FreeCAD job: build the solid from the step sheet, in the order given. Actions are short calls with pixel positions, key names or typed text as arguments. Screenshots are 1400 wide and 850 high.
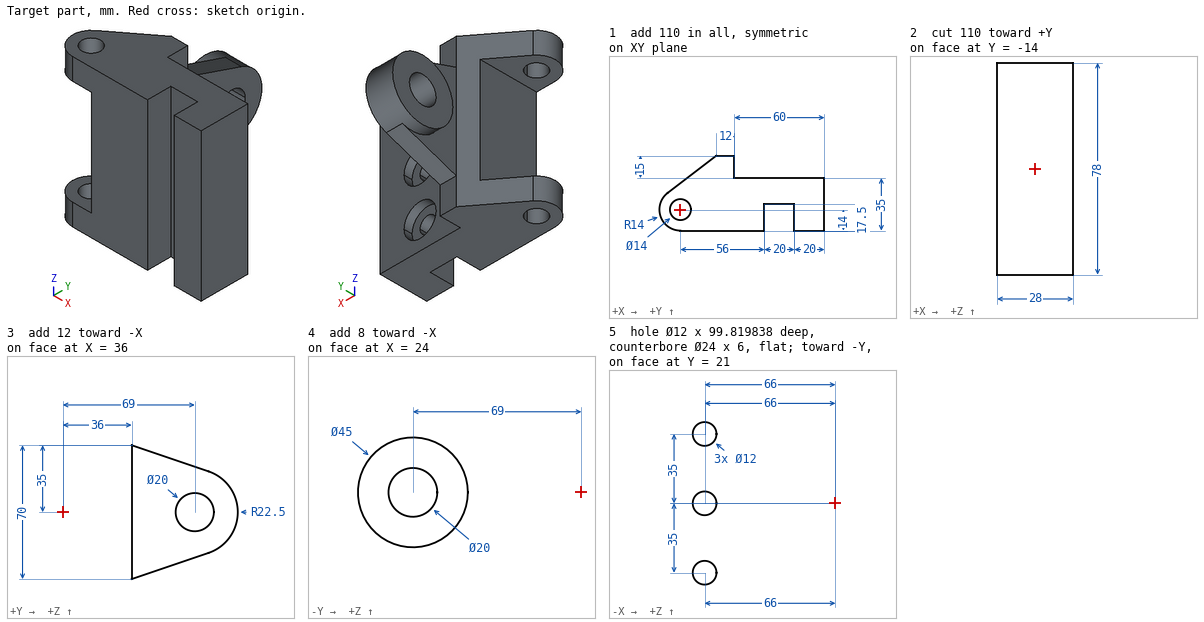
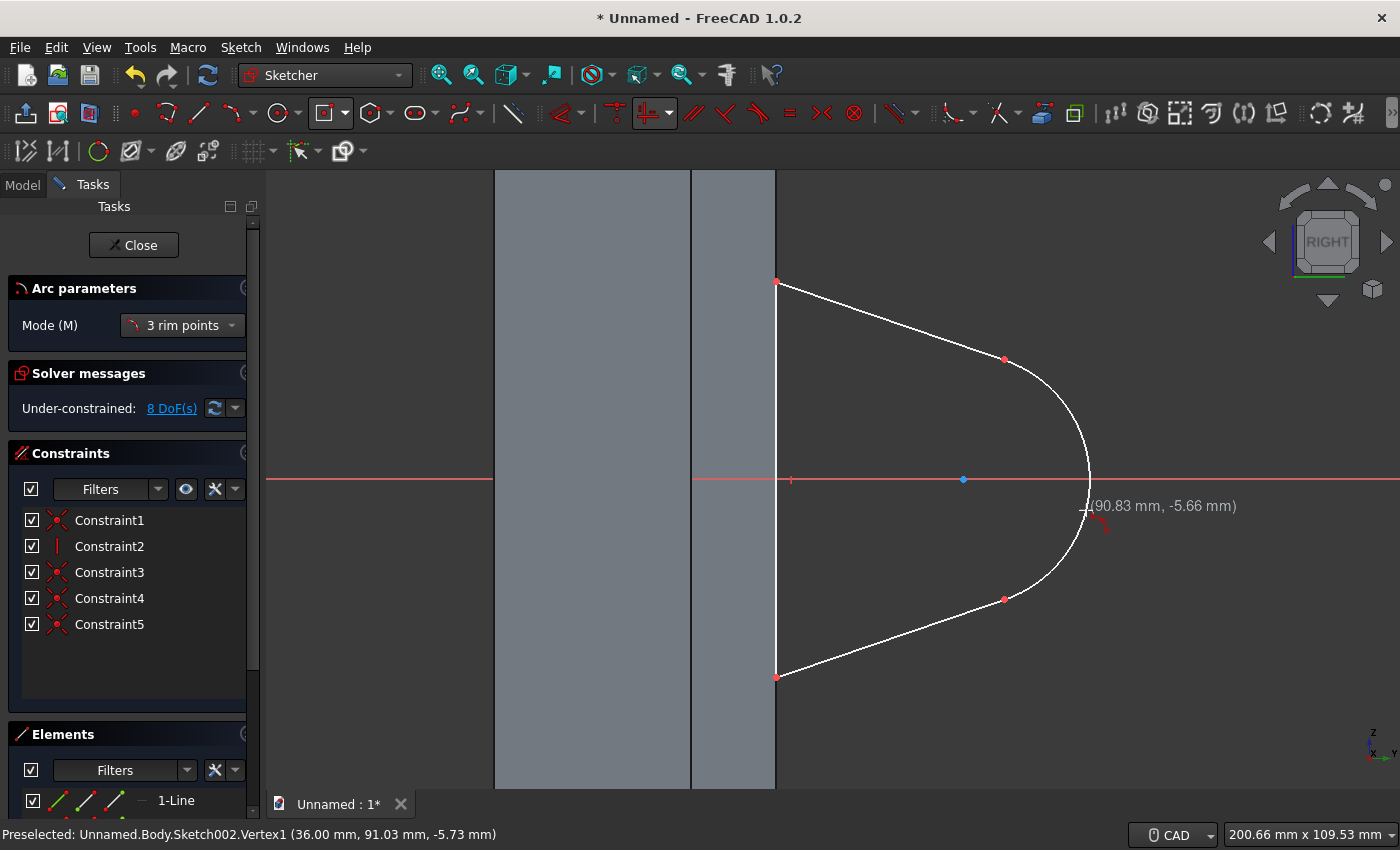
click(278, 114)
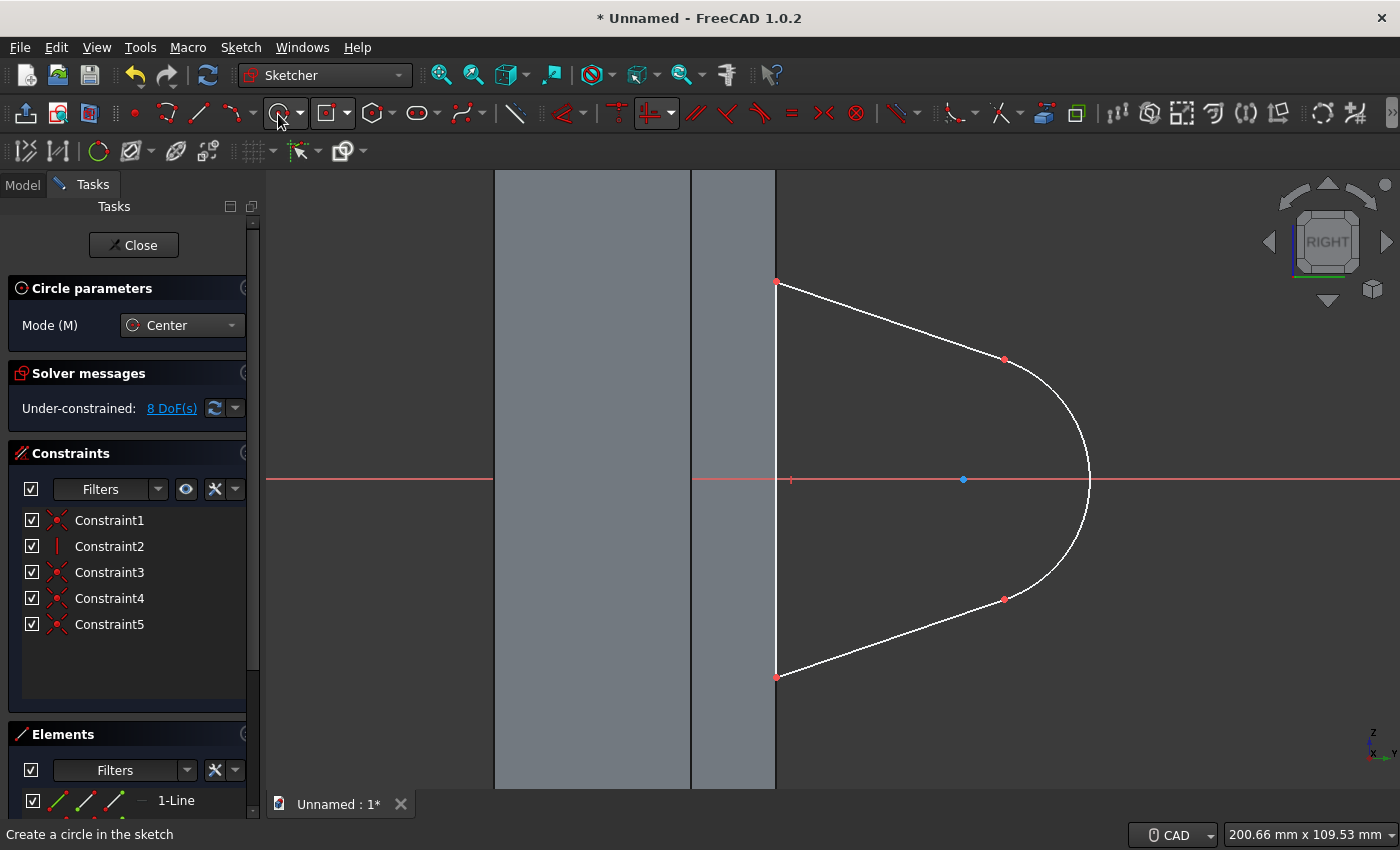
click(963, 479)
click(1003, 439)
key(Escape)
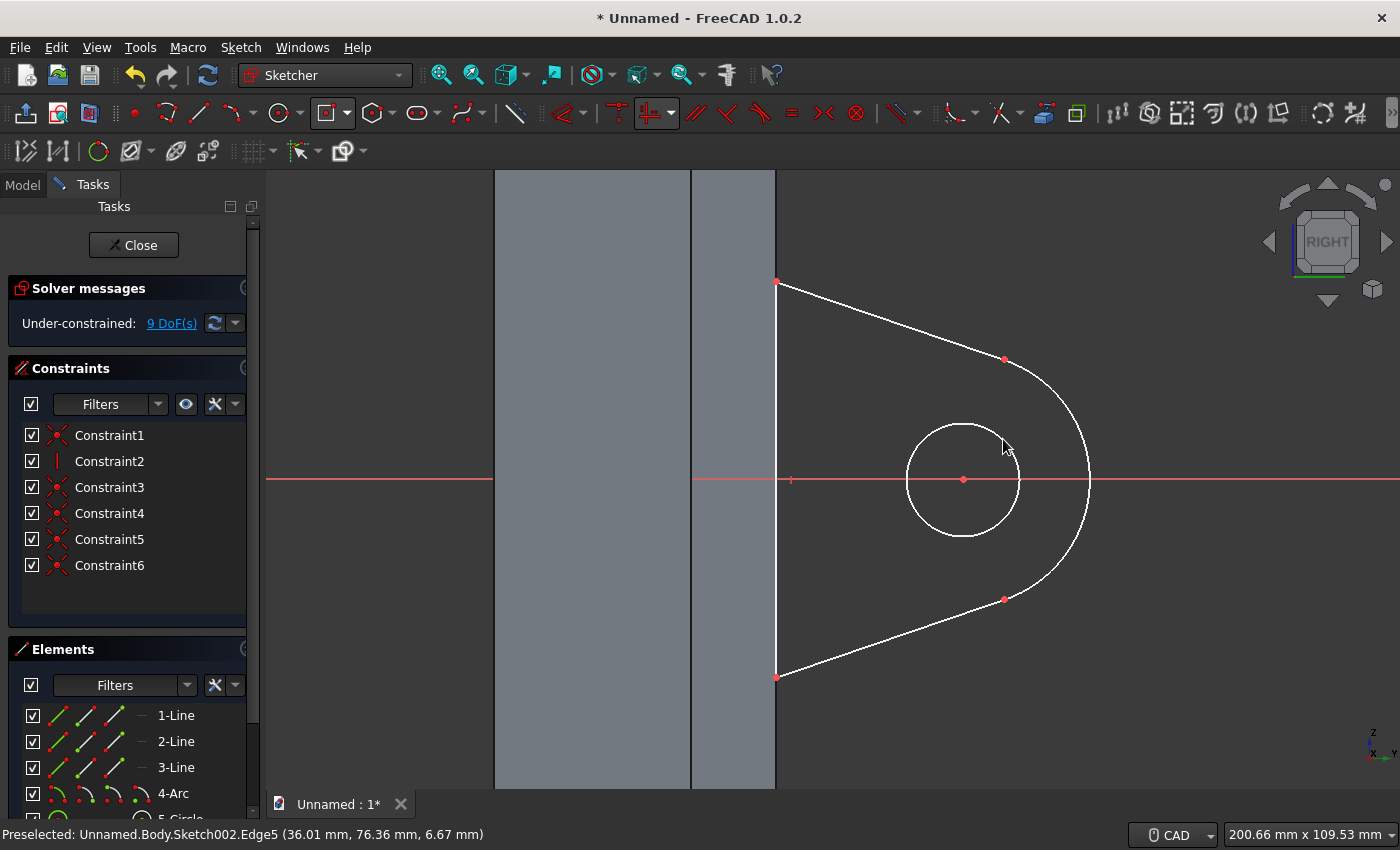
click(936, 337)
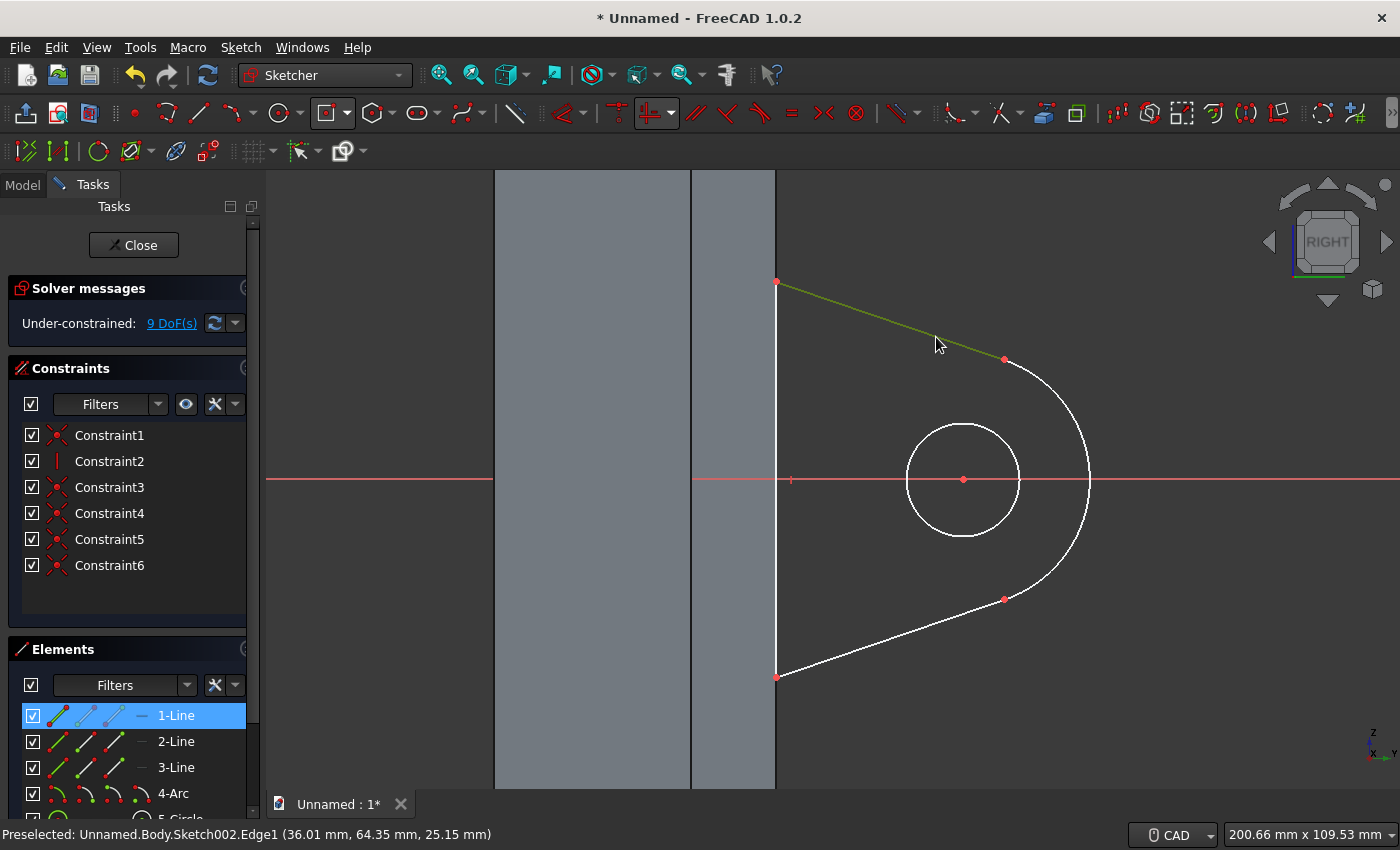
click(1075, 540)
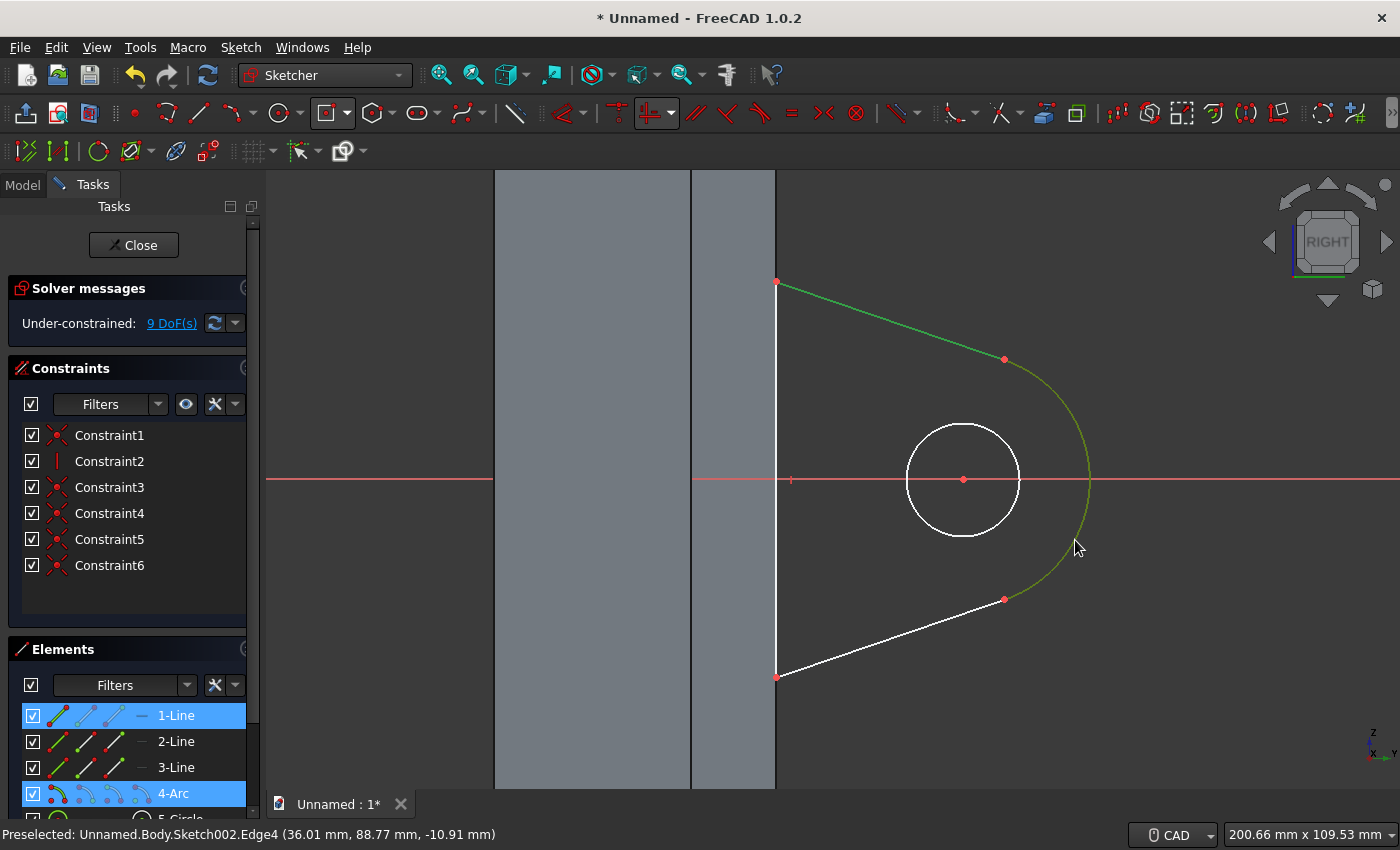
click(760, 114)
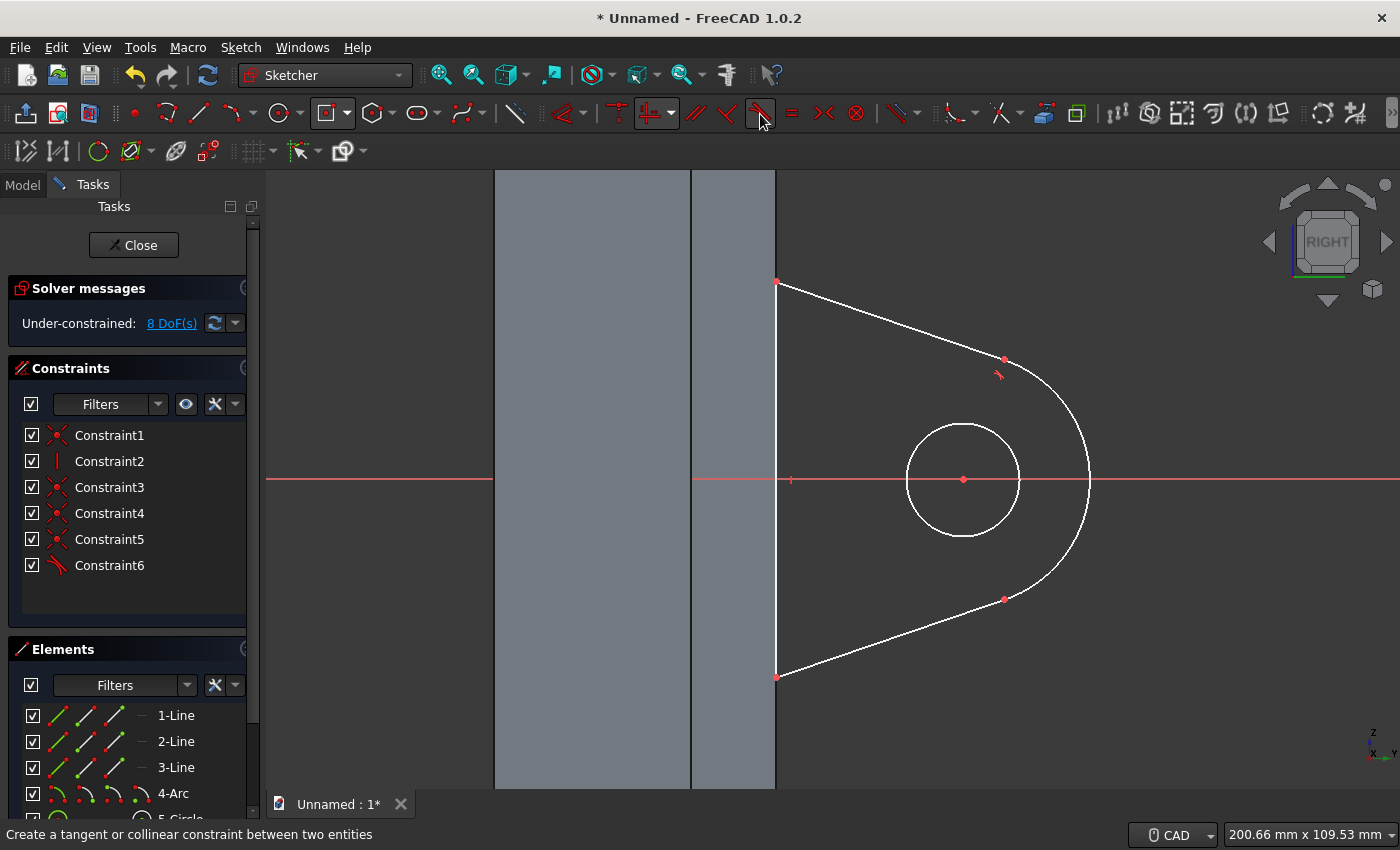
click(844, 655)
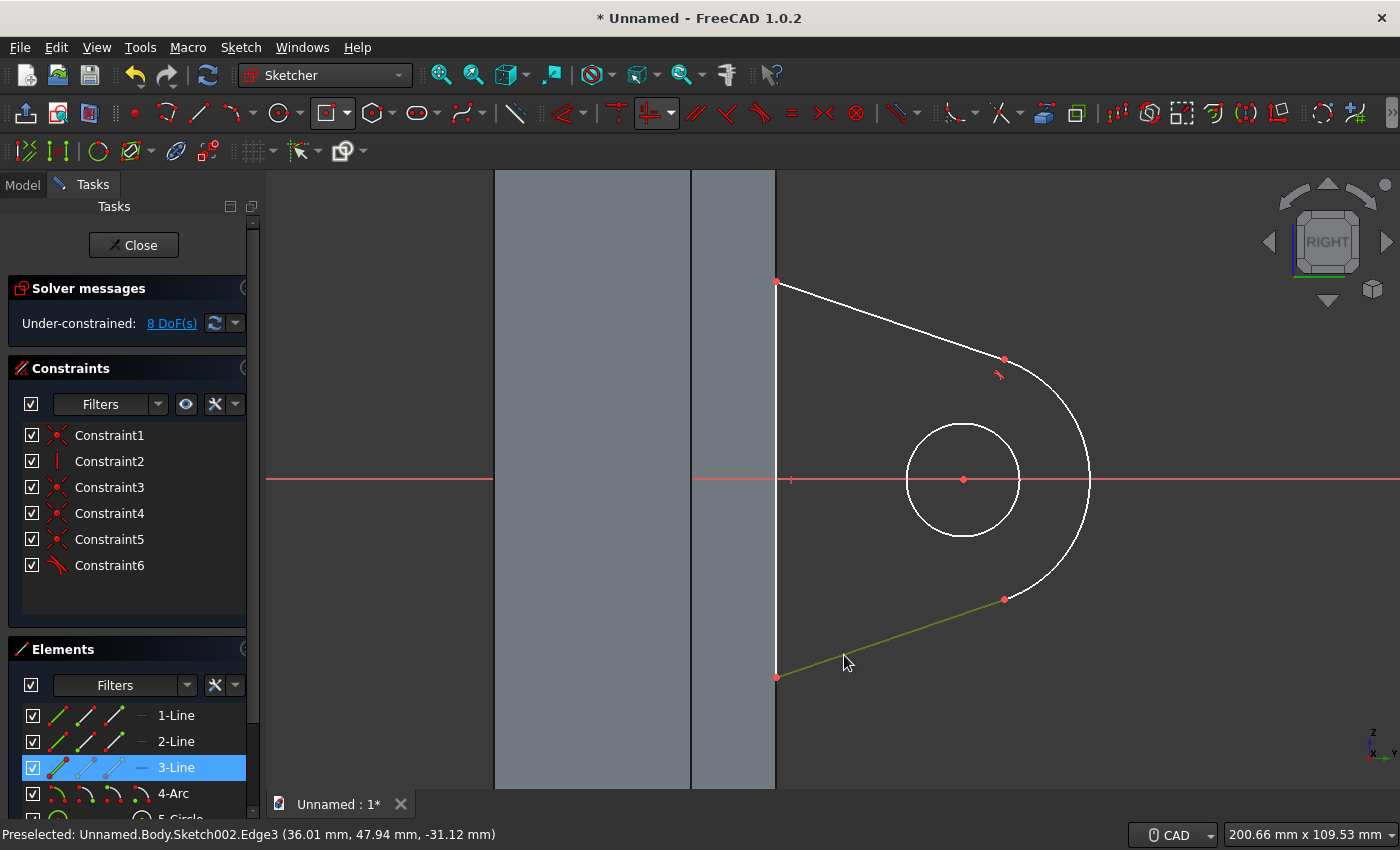
click(1075, 540)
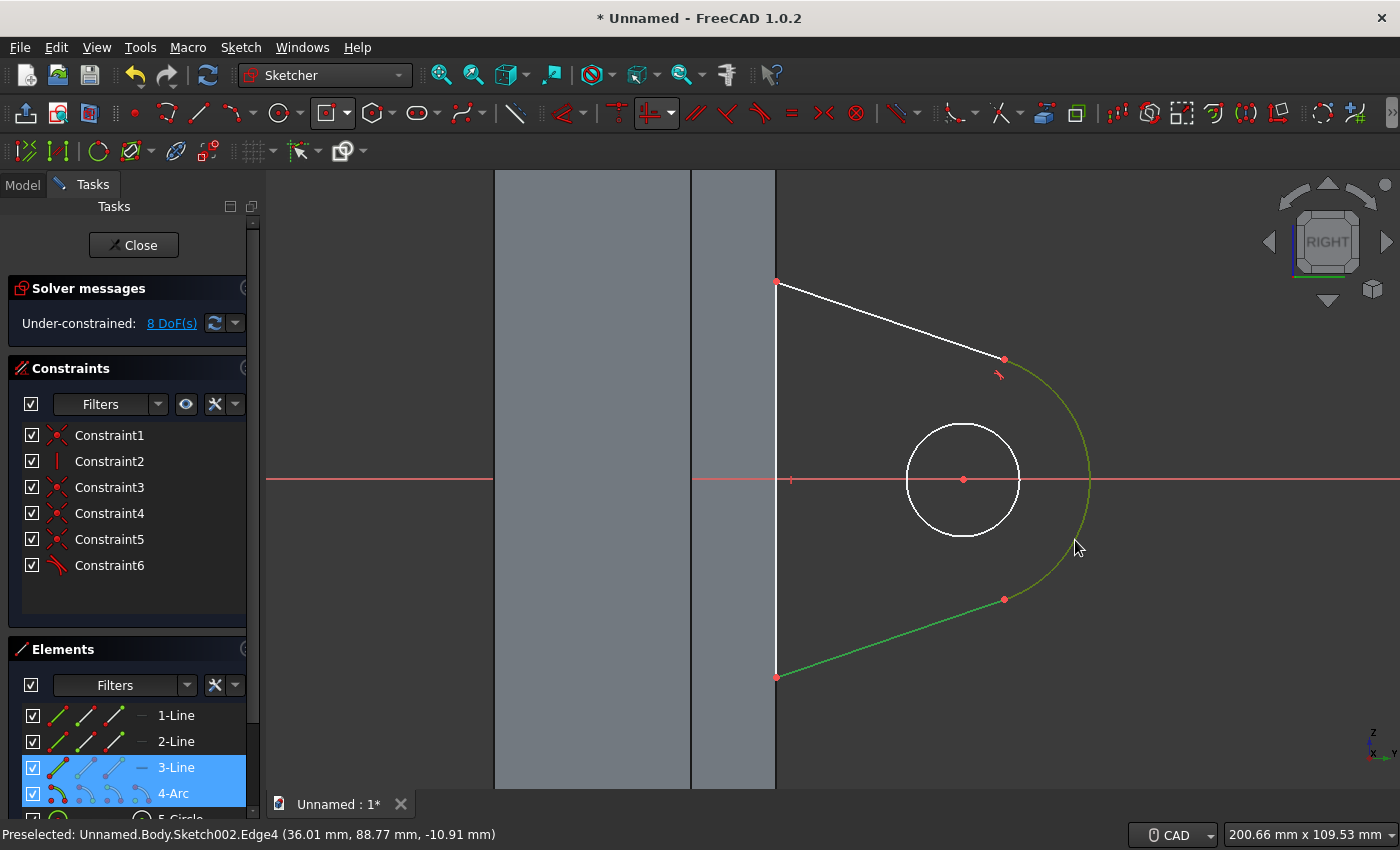
click(760, 114)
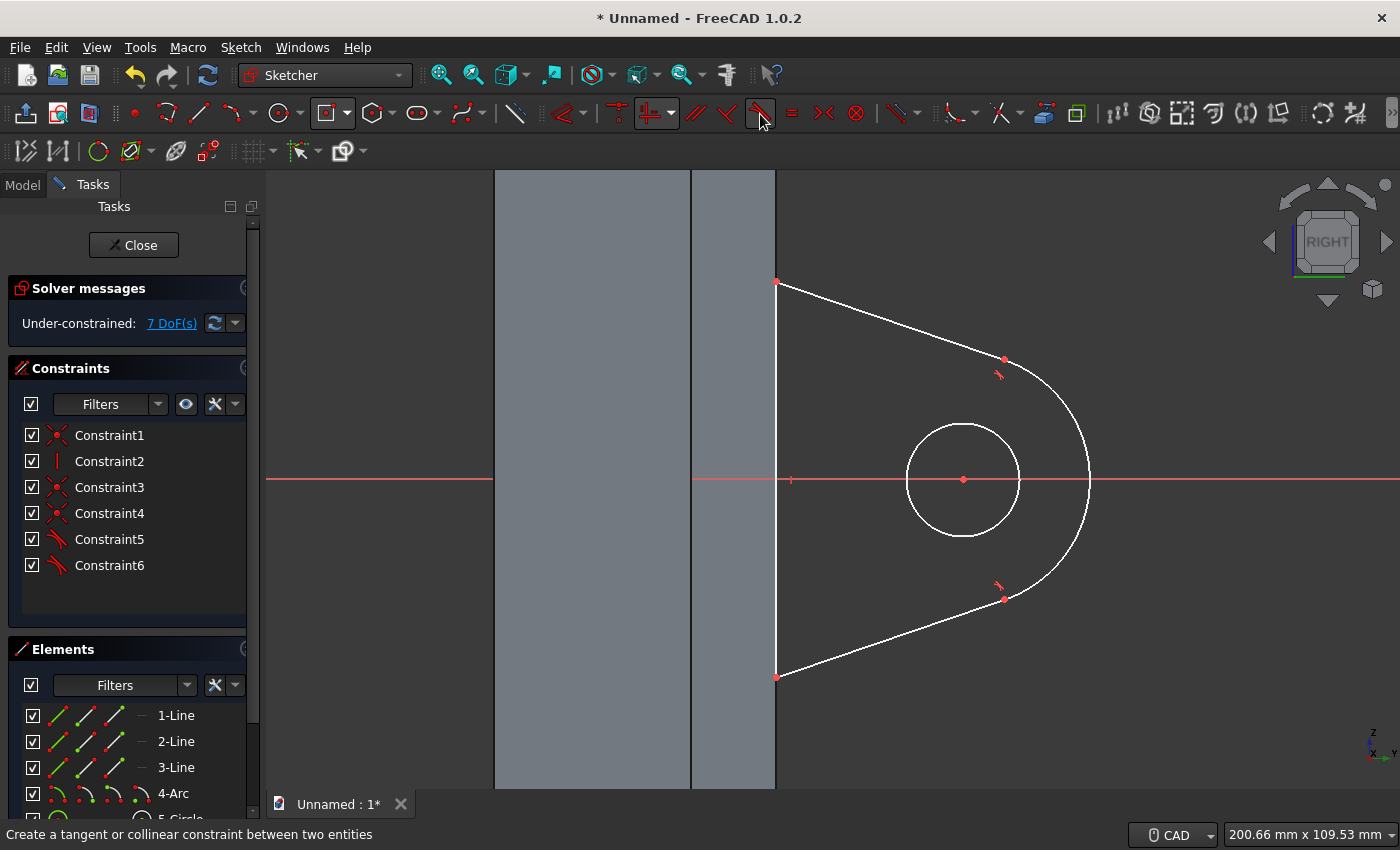
click(963, 480)